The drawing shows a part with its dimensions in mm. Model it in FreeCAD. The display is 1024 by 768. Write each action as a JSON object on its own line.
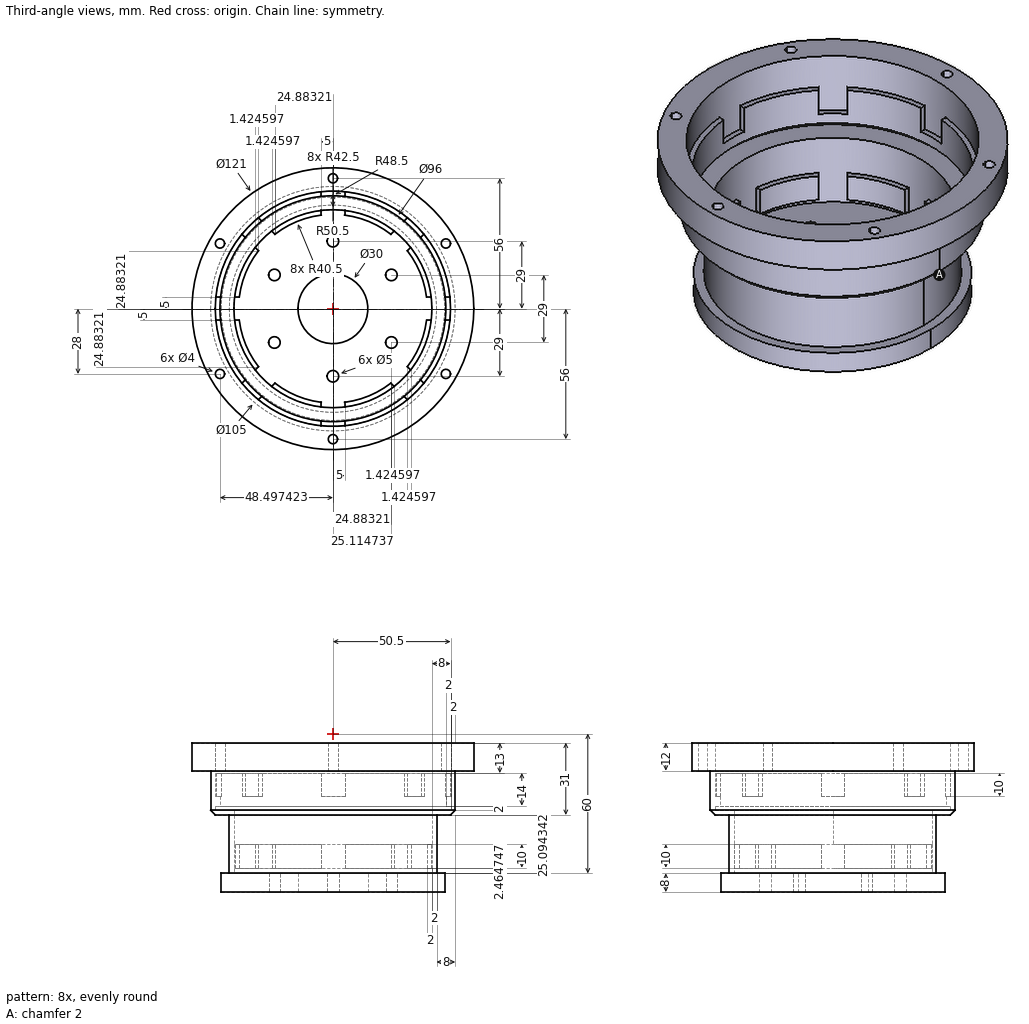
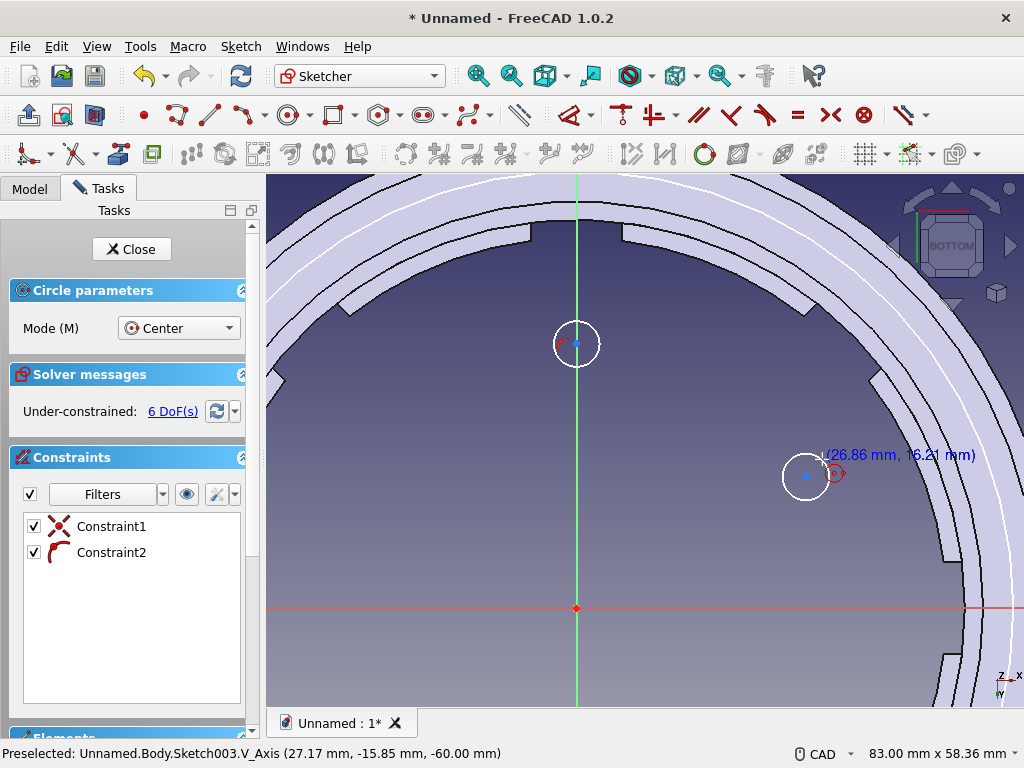
{"action": "left_click", "coordinate": [347, 476]}
{"action": "left_click", "coordinate": [364, 459]}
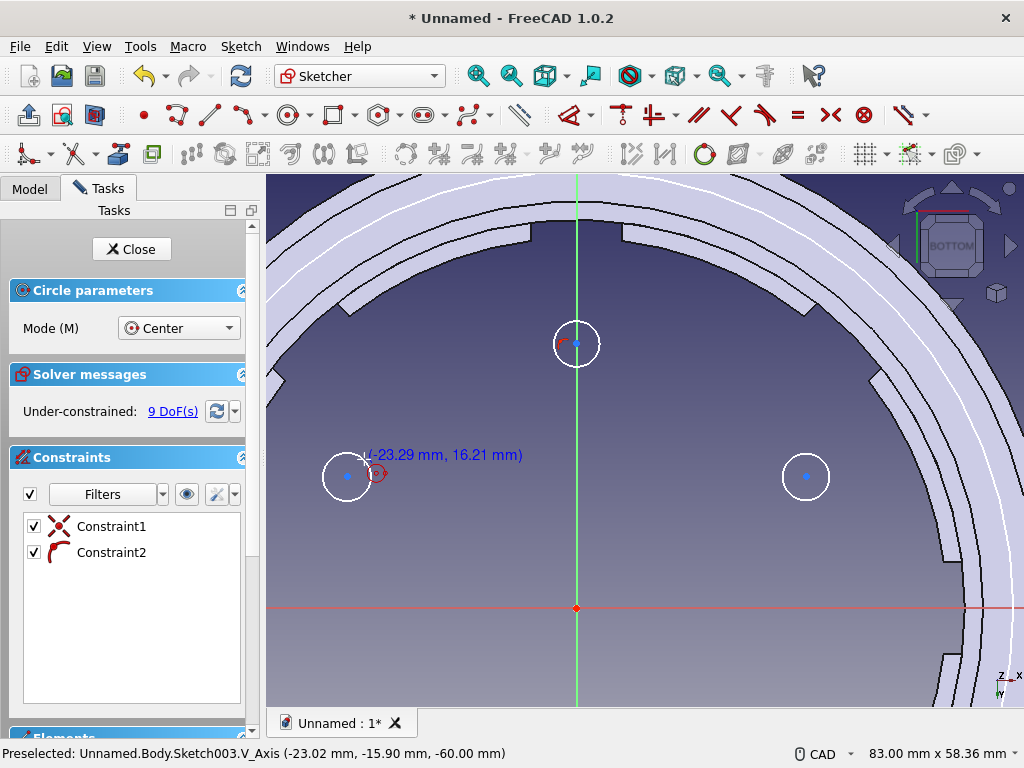
{"action": "scroll", "coordinate": [576, 343], "scroll_direction": "down", "scroll_amount": 5}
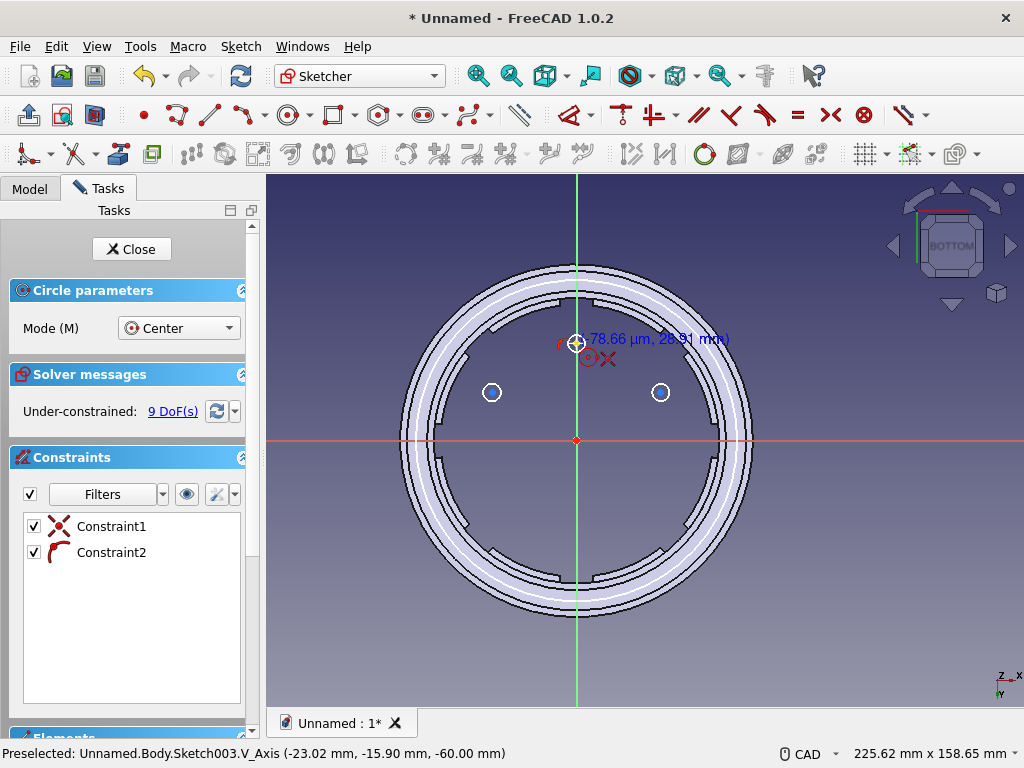
{"action": "scroll", "coordinate": [661, 489], "scroll_direction": "up", "scroll_amount": 5}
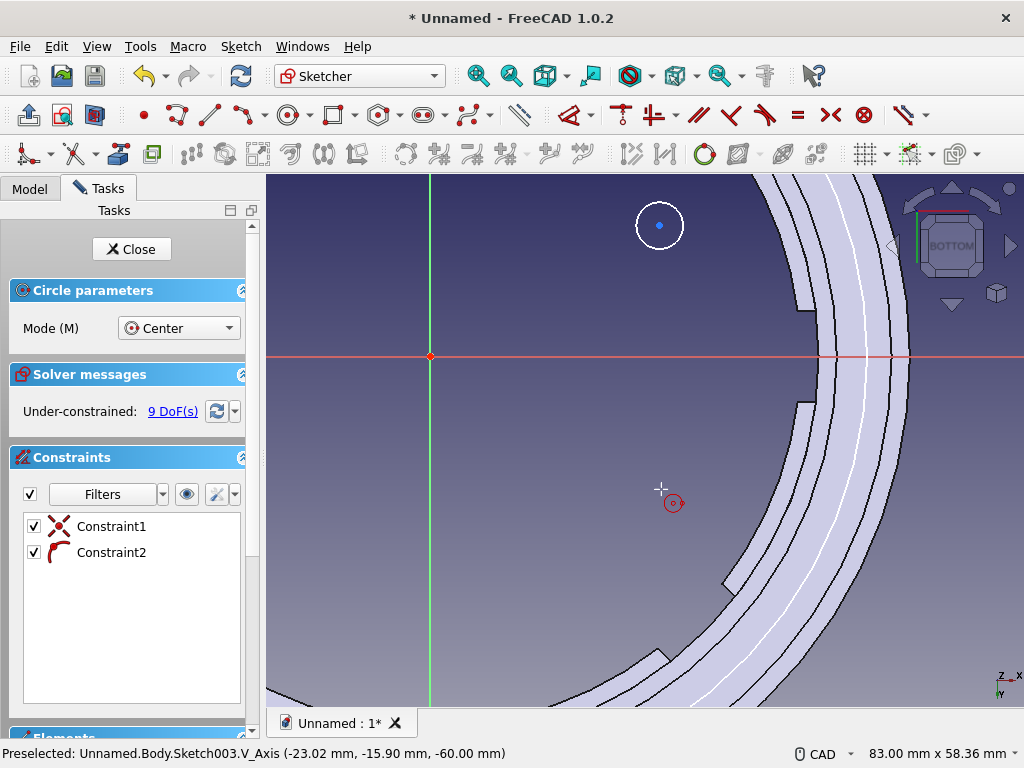
{"action": "left_click", "coordinate": [660, 489]}
{"action": "left_click", "coordinate": [676, 473]}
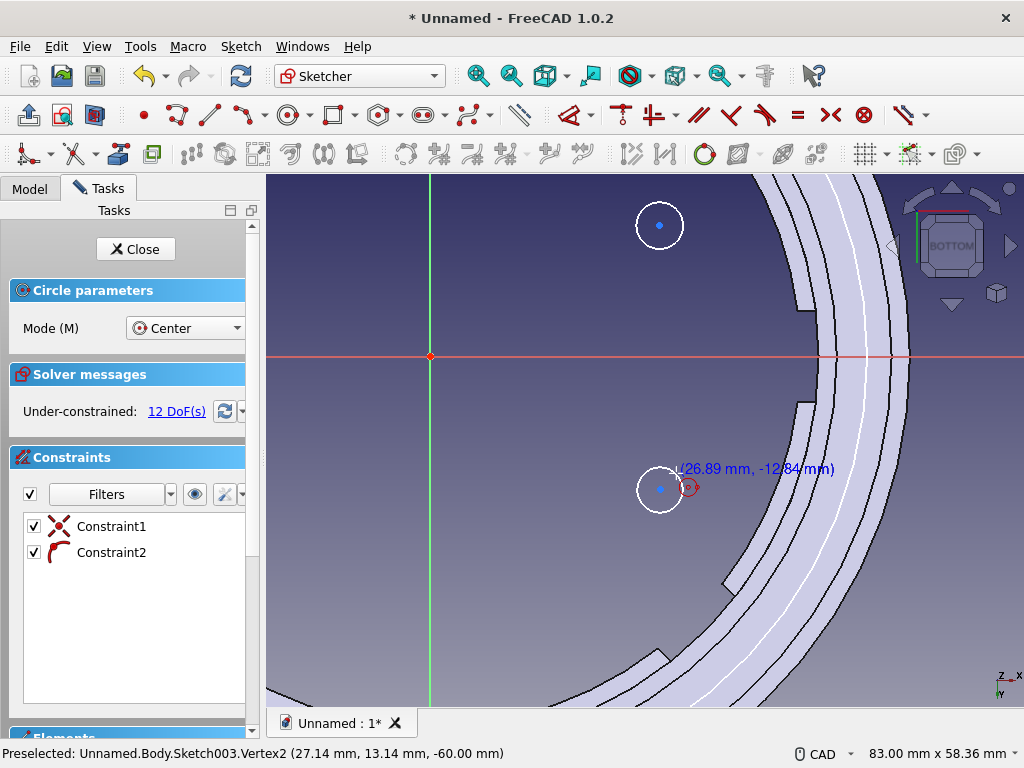
{"action": "left_click", "coordinate": [430, 357]}
{"action": "left_click", "coordinate": [527, 260]}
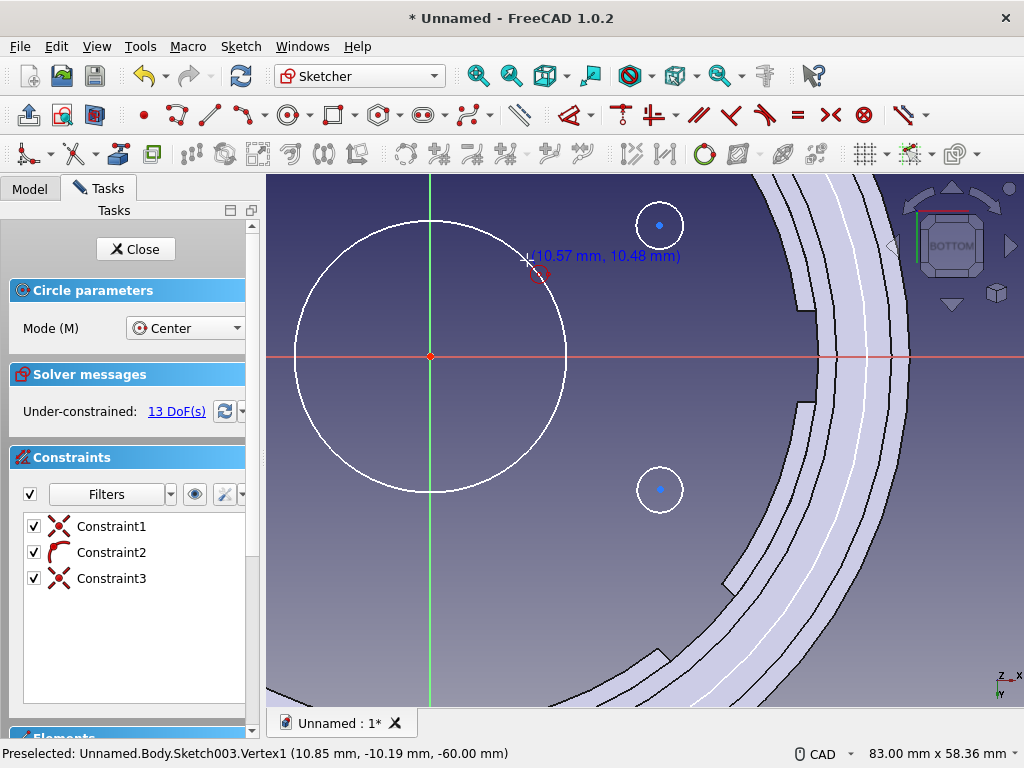
{"action": "left_click", "coordinate": [430, 622]}
{"action": "left_click", "coordinate": [447, 605]}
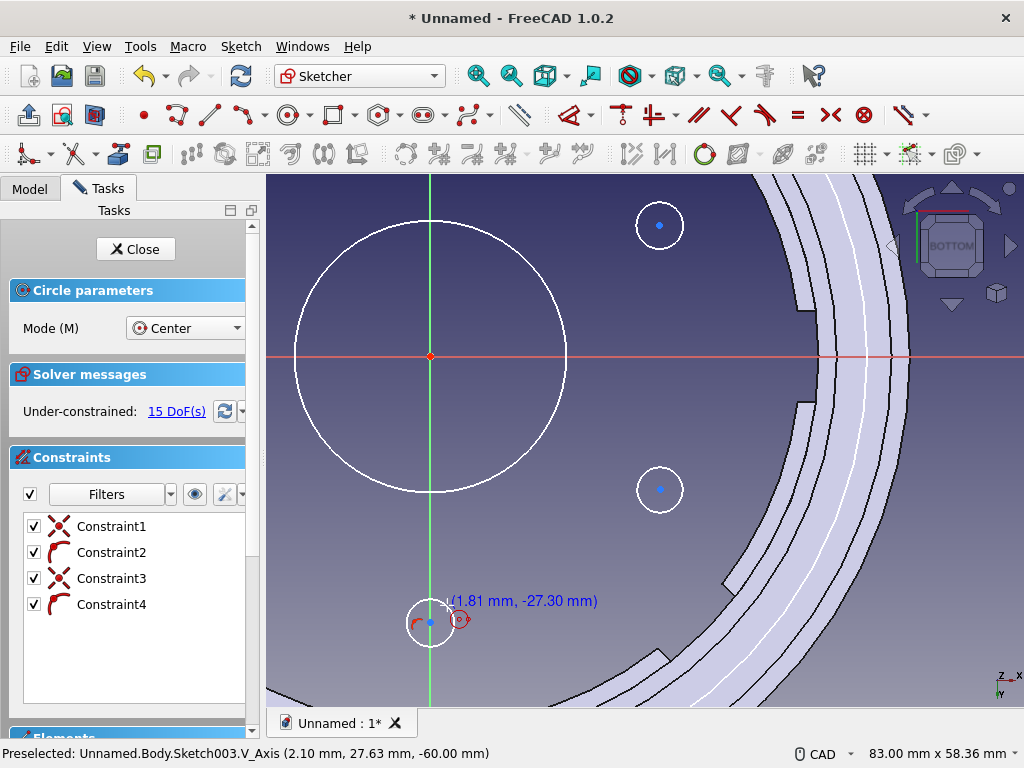
{"action": "scroll", "coordinate": [661, 489], "scroll_direction": "down", "scroll_amount": 5}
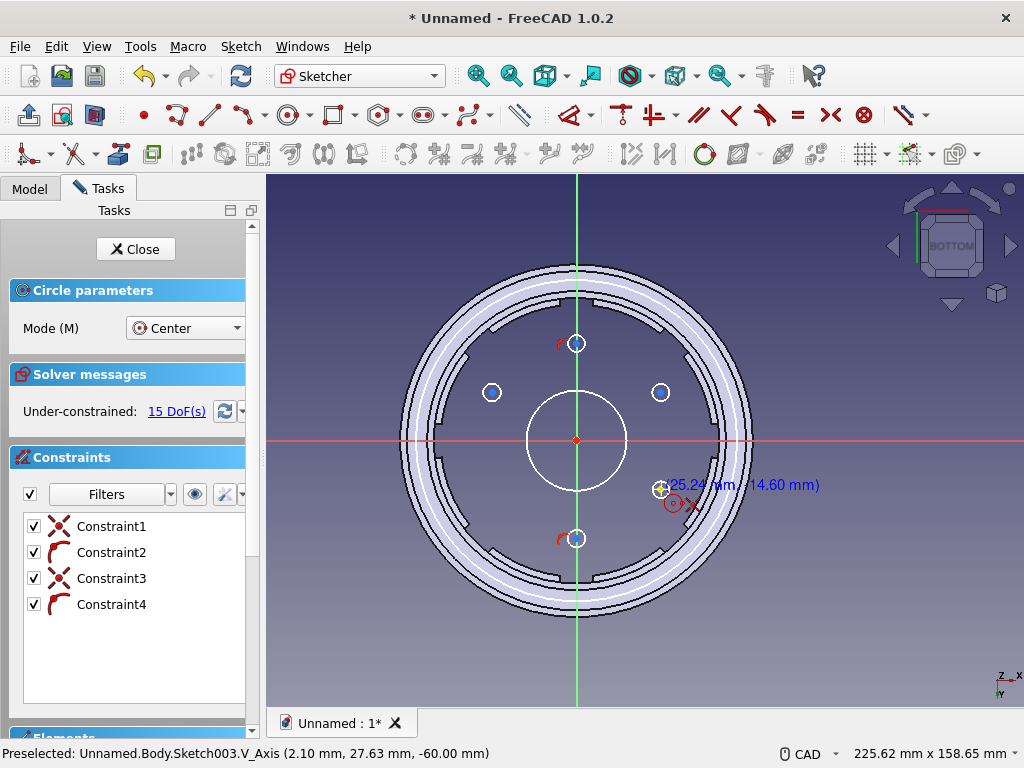
{"action": "scroll", "coordinate": [492, 489], "scroll_direction": "up", "scroll_amount": 5}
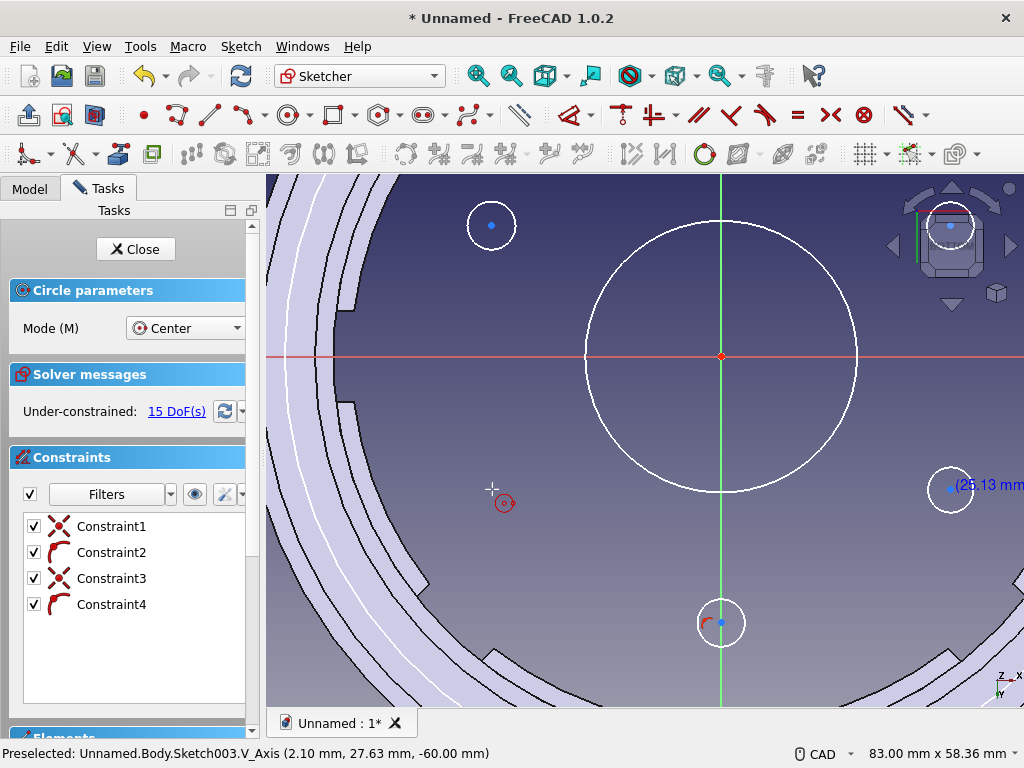
{"action": "left_click", "coordinate": [492, 489]}
{"action": "left_click", "coordinate": [508, 473]}
{"action": "key", "text": "Escape"}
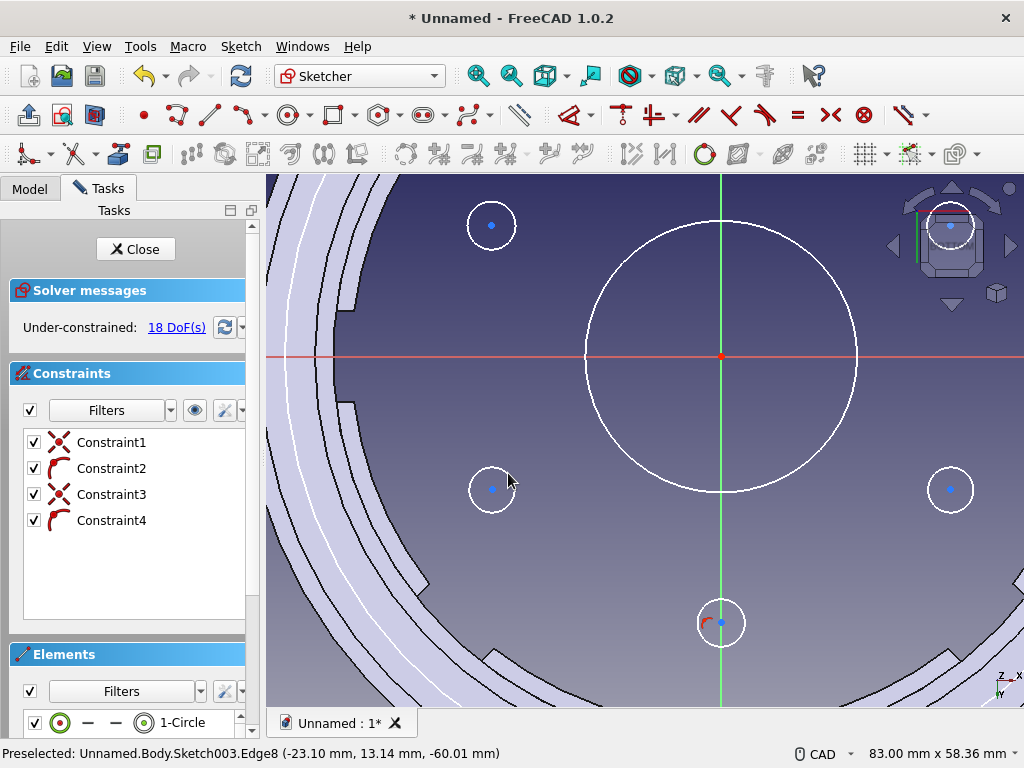
{"action": "scroll", "coordinate": [492, 489], "scroll_direction": "down", "scroll_amount": 5}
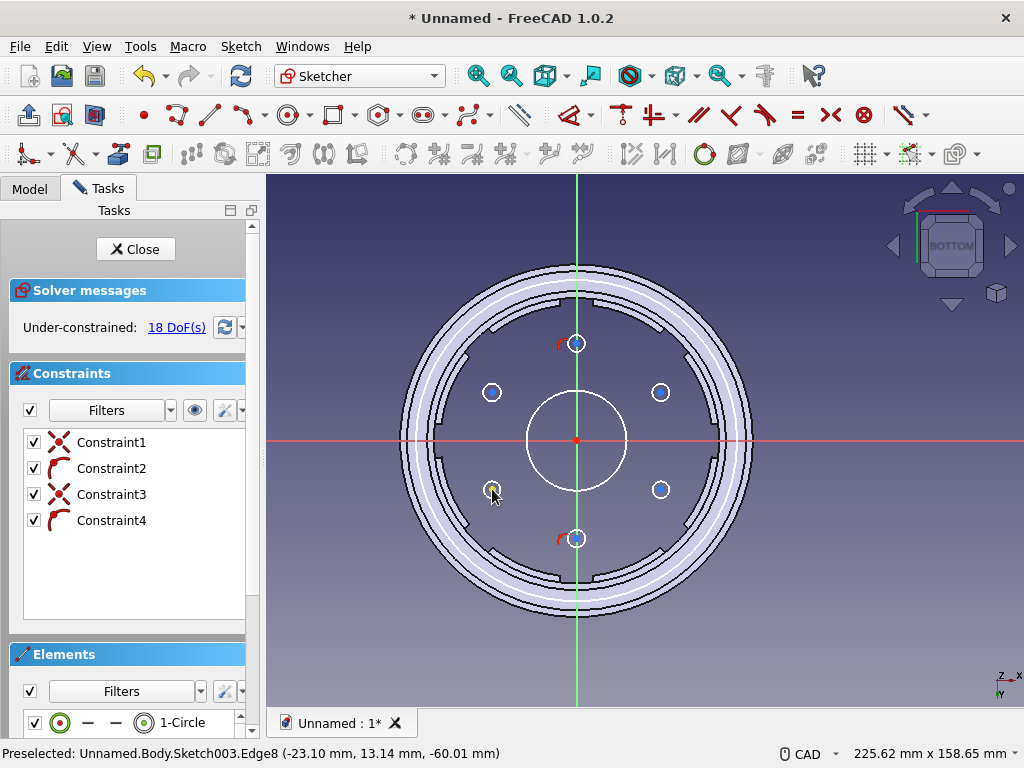
{"action": "scroll", "coordinate": [582, 338], "scroll_direction": "up", "scroll_amount": 5}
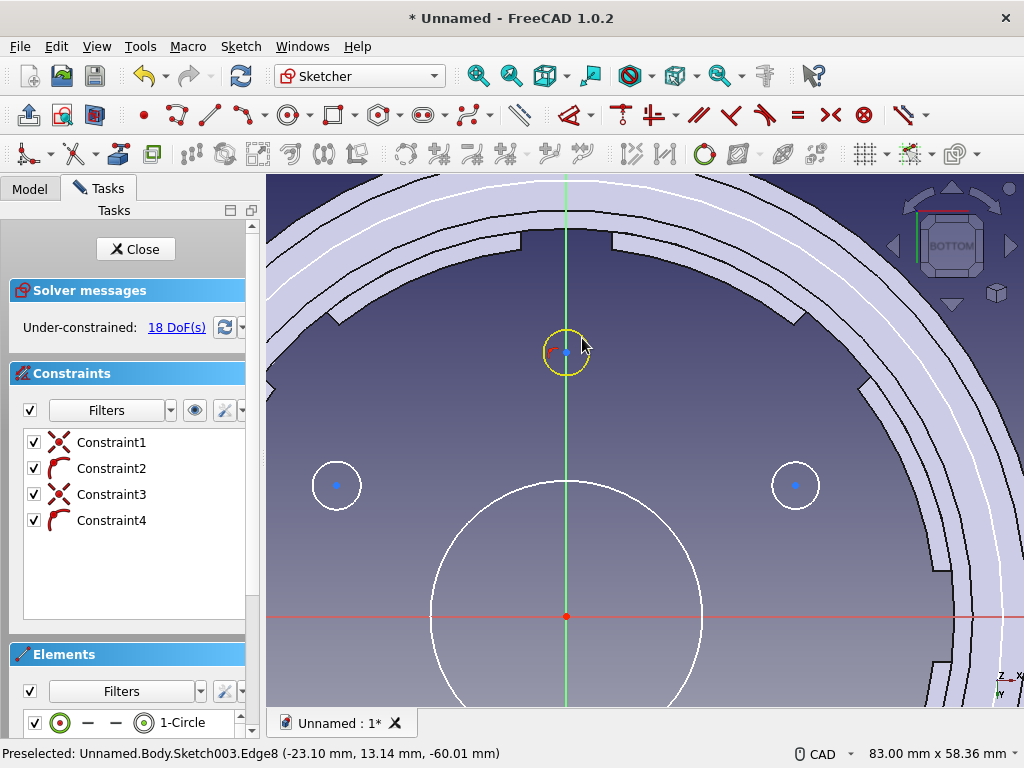
{"action": "left_click", "coordinate": [582, 336]}